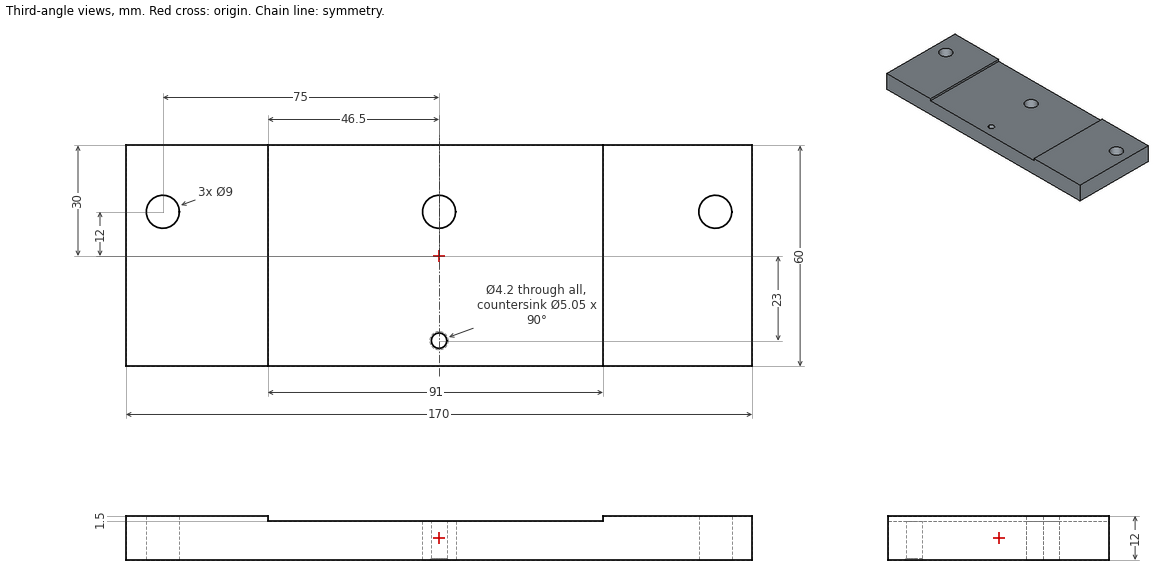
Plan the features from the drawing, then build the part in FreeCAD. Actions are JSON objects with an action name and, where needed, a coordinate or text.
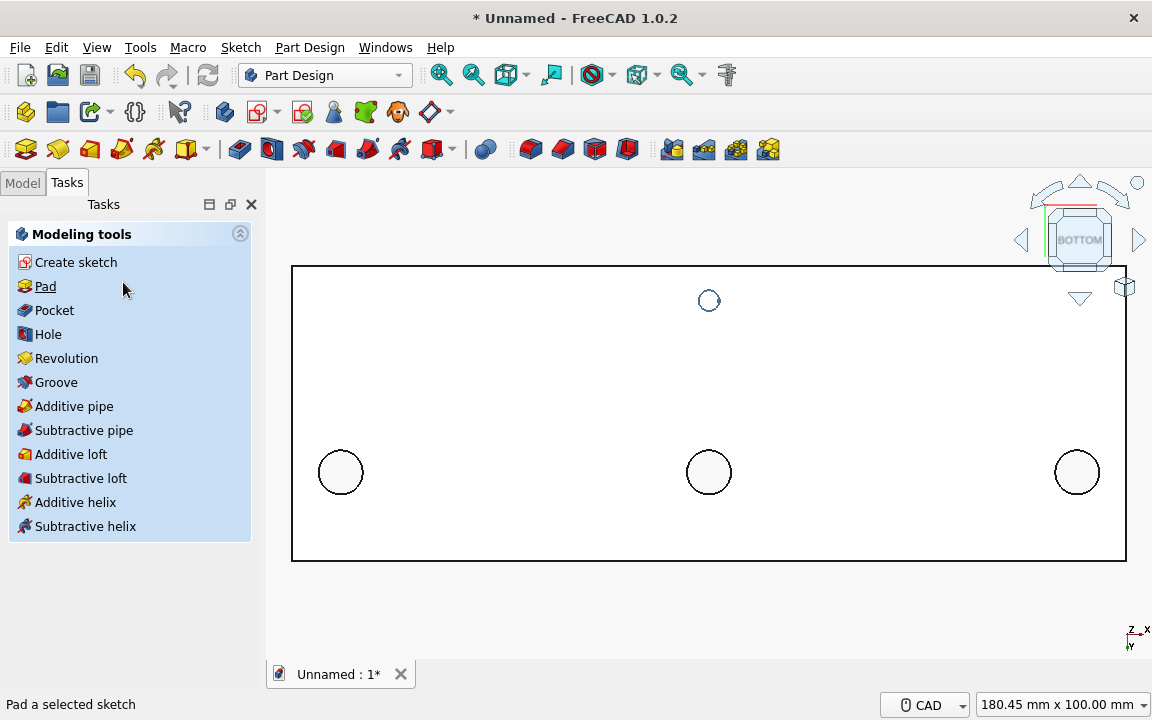
{"action": "left_click", "coordinate": [272, 150]}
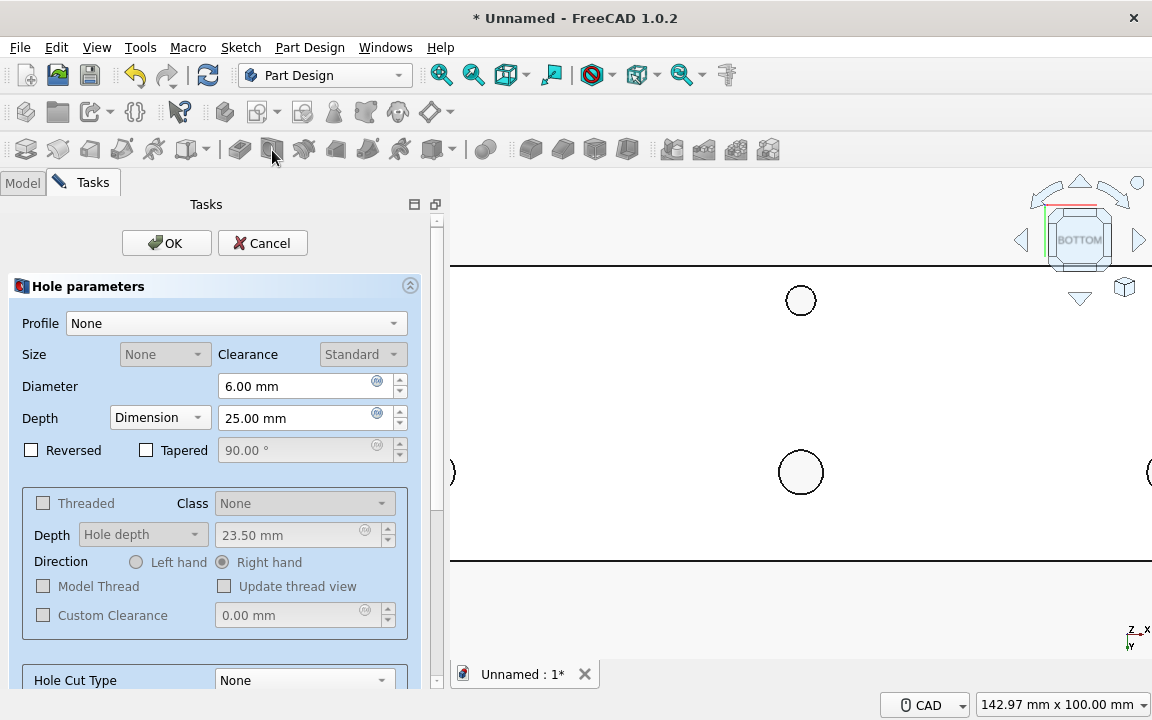
{"action": "triple_click", "coordinate": [305, 386]}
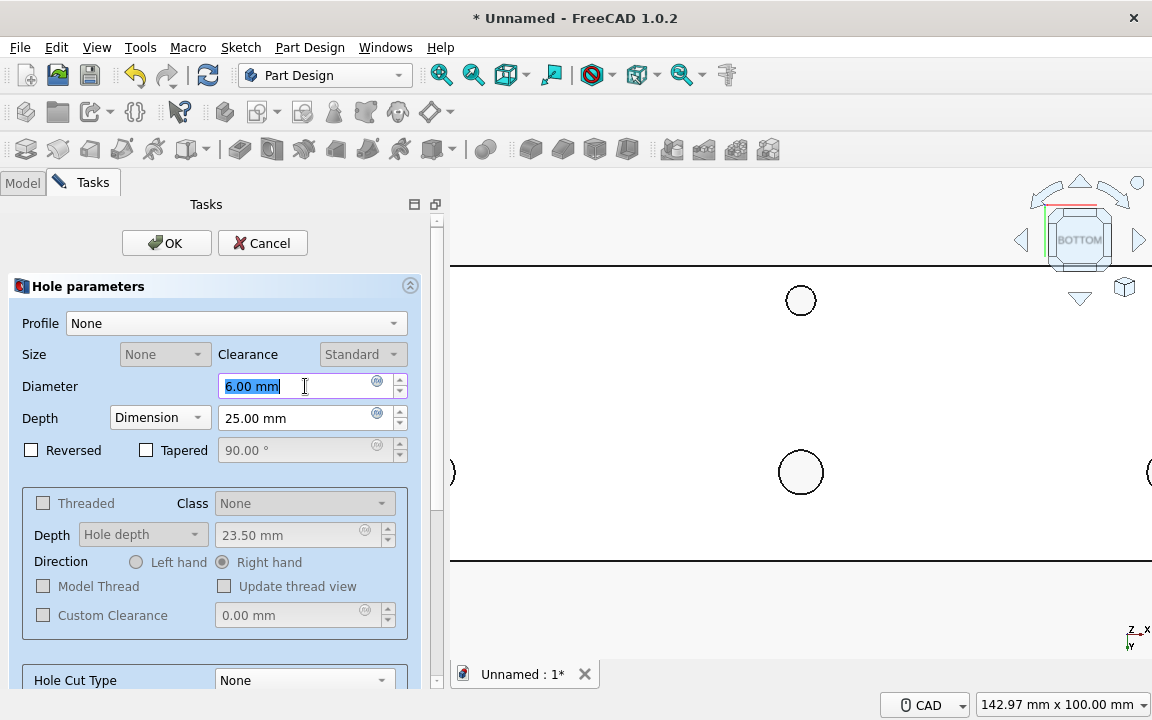
{"action": "type", "text": "4.2"}
{"action": "key", "text": "Tab"}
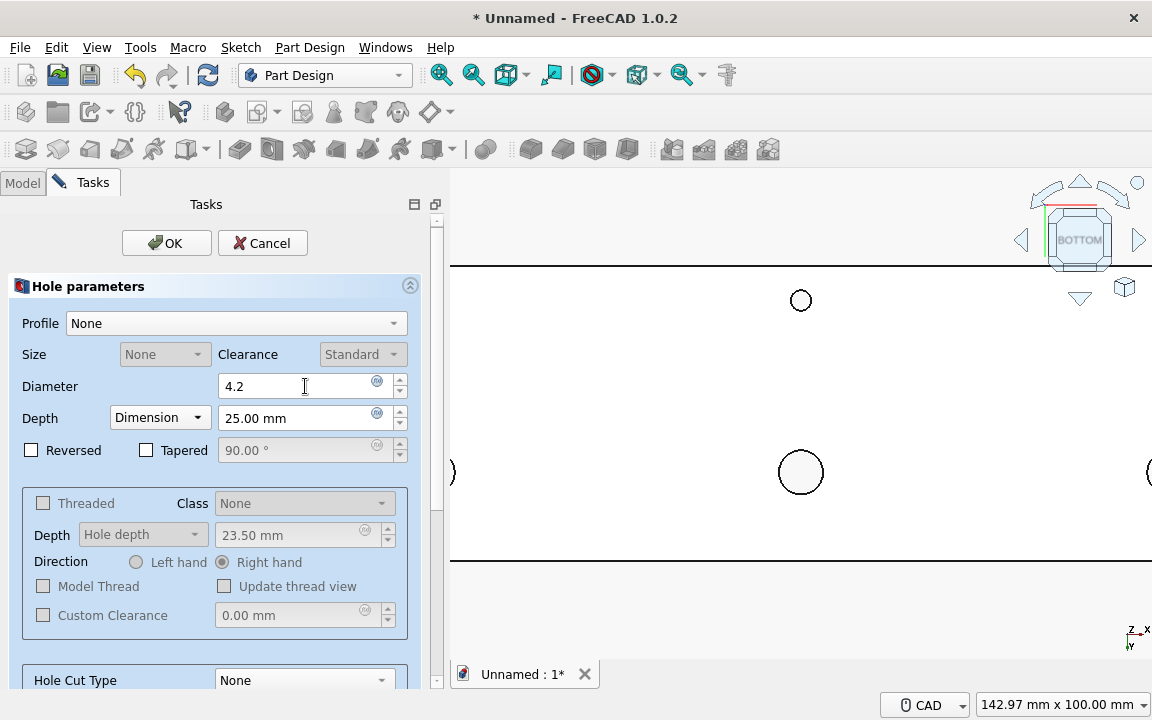
{"action": "left_click", "coordinate": [161, 418]}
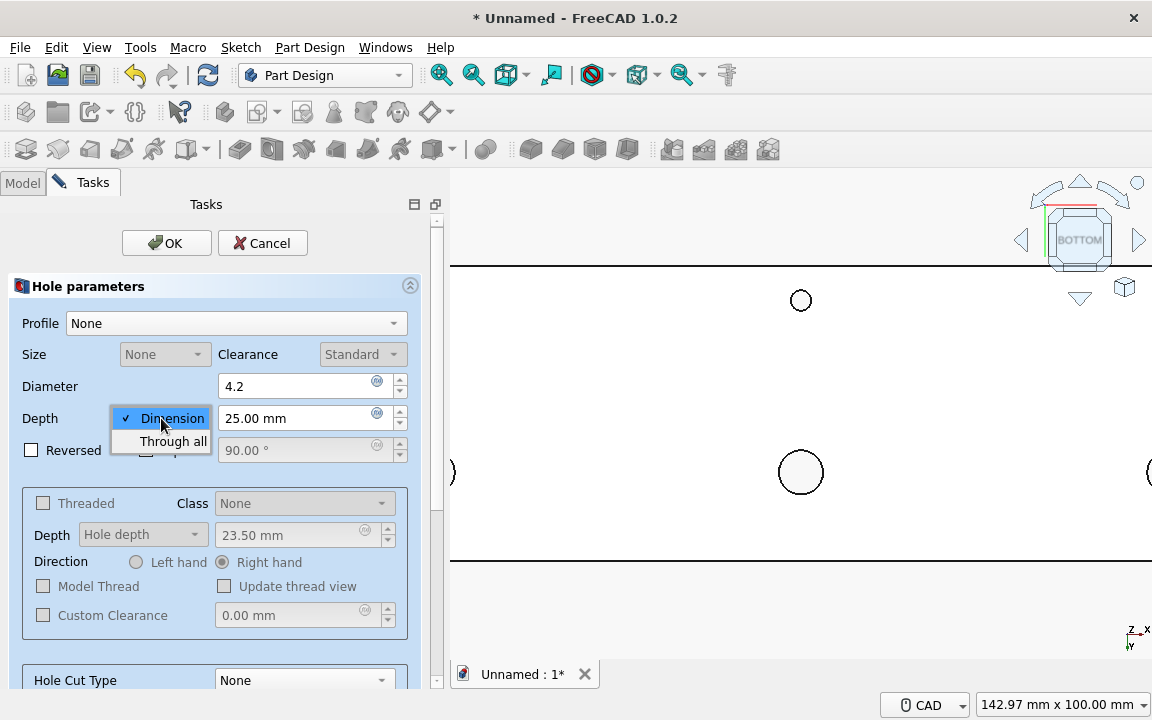
{"action": "left_click", "coordinate": [160, 442]}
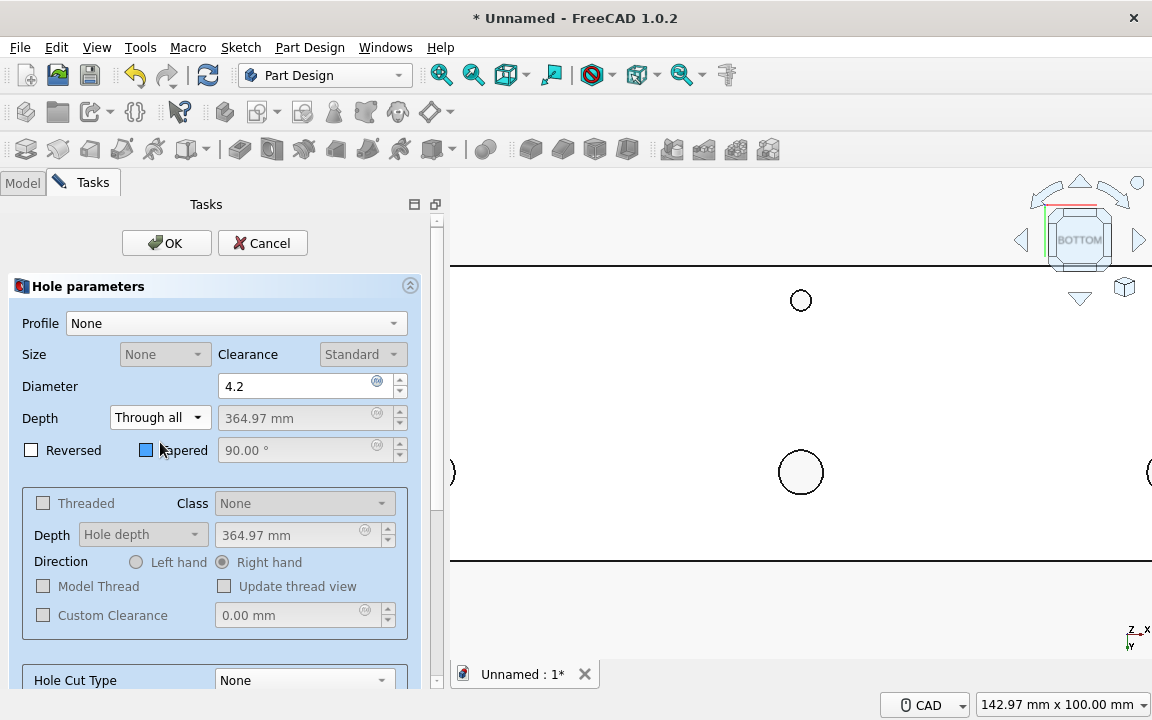
{"action": "scroll", "coordinate": [437, 451], "scroll_direction": "down", "scroll_amount": 2}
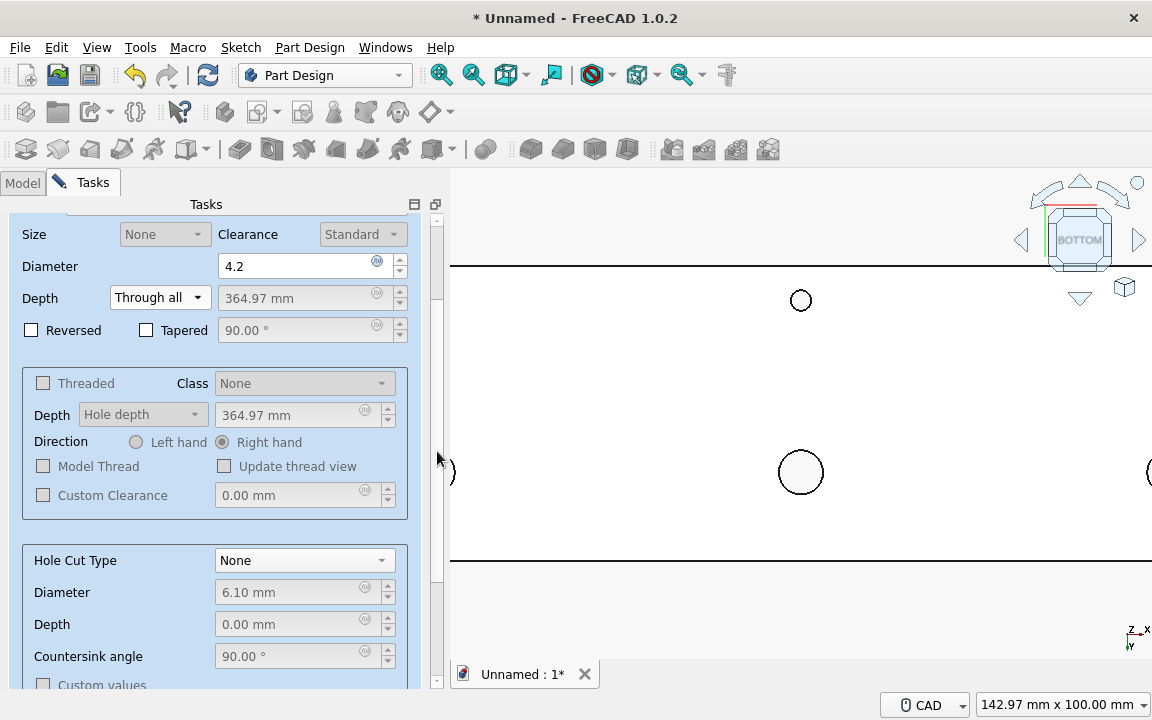
{"action": "left_click", "coordinate": [306, 560]}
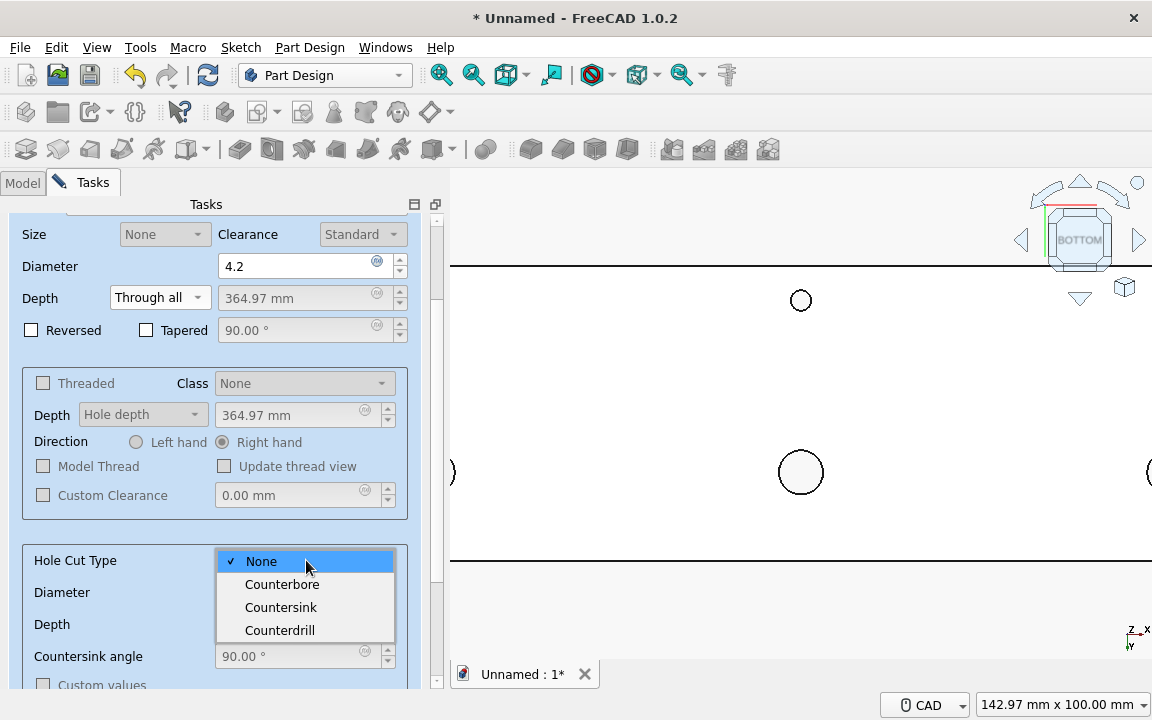
{"action": "left_click", "coordinate": [304, 608]}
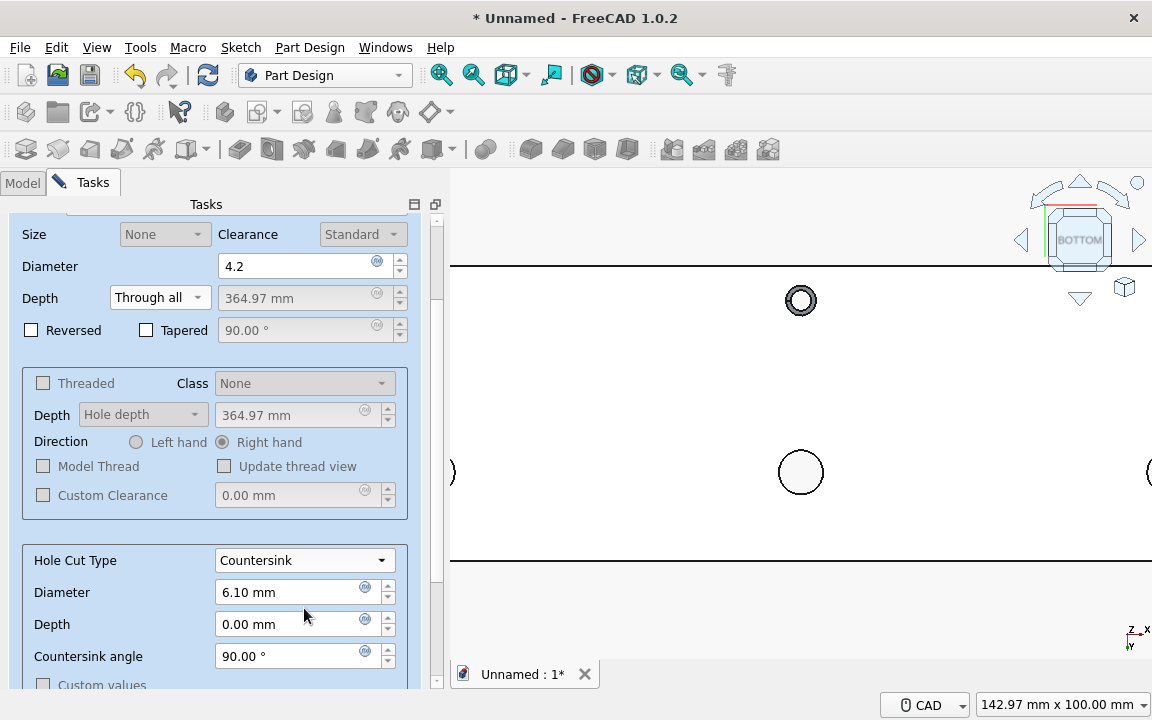
{"action": "triple_click", "coordinate": [298, 592]}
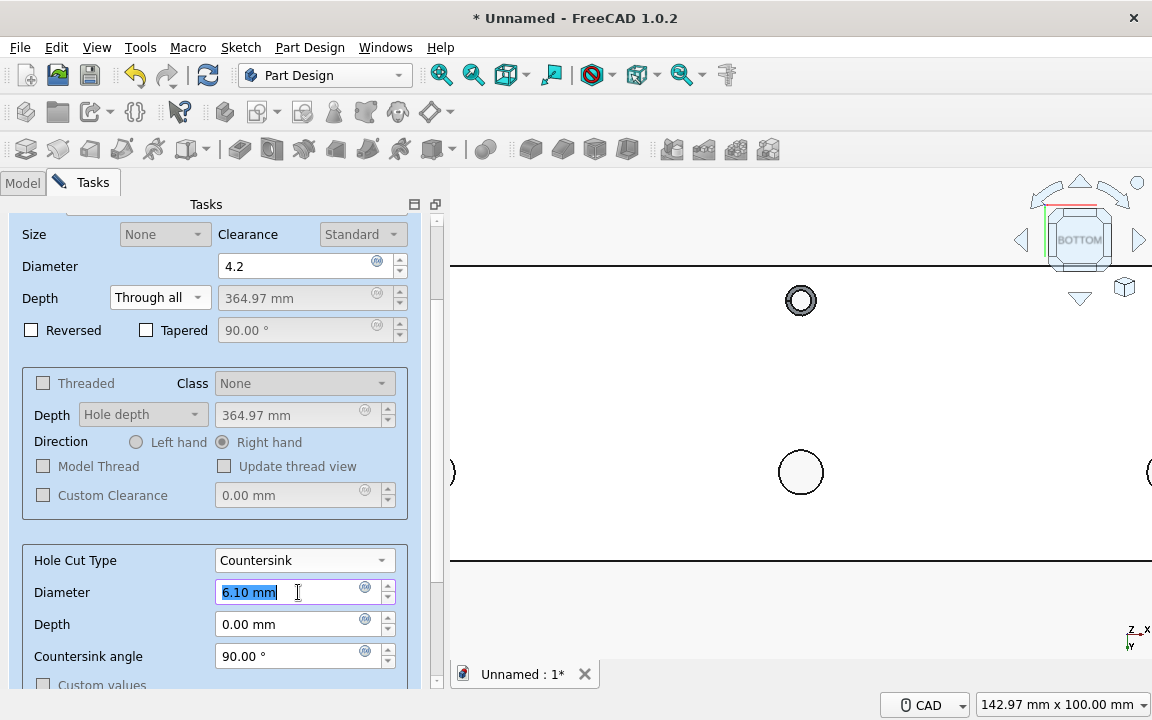
{"action": "type", "text": "5.05"}
{"action": "key", "text": "Tab"}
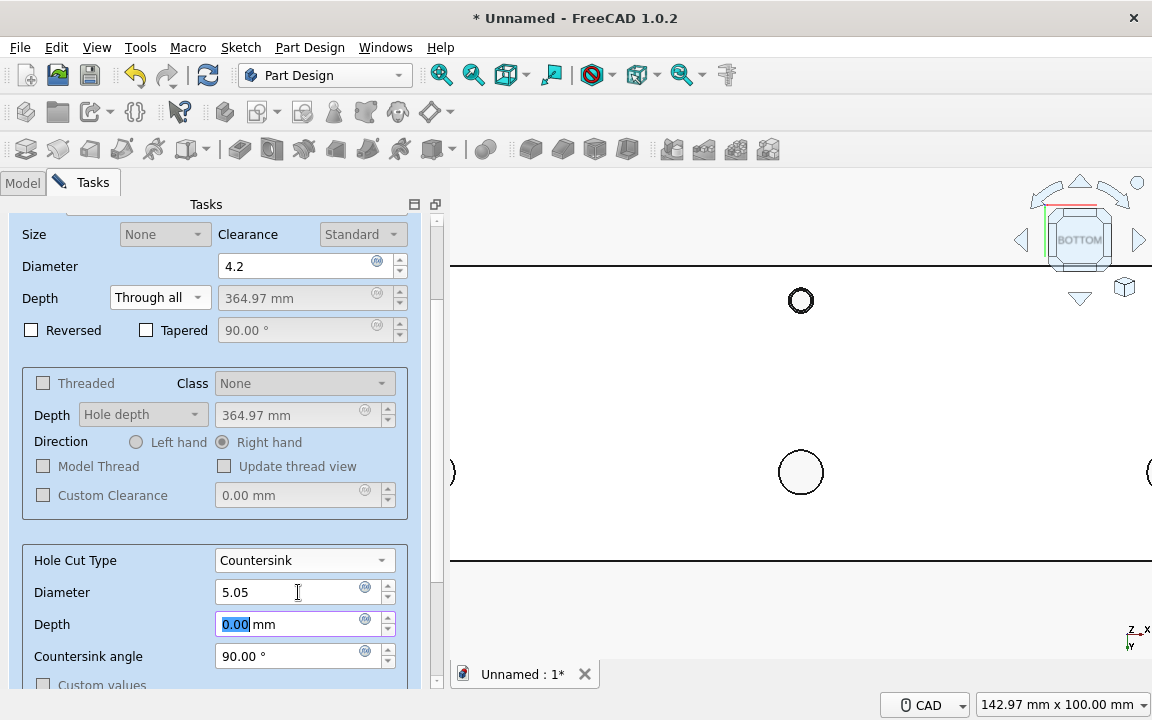
{"action": "scroll", "coordinate": [437, 451], "scroll_direction": "up", "scroll_amount": 3}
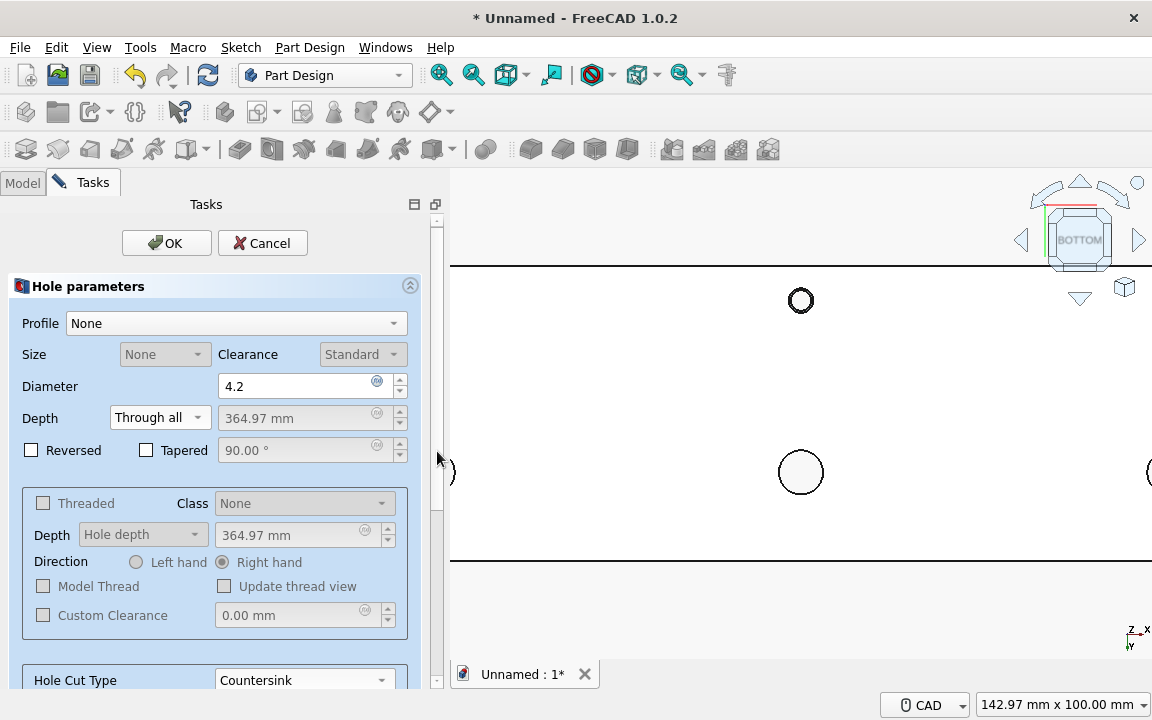
{"action": "left_click", "coordinate": [167, 243]}